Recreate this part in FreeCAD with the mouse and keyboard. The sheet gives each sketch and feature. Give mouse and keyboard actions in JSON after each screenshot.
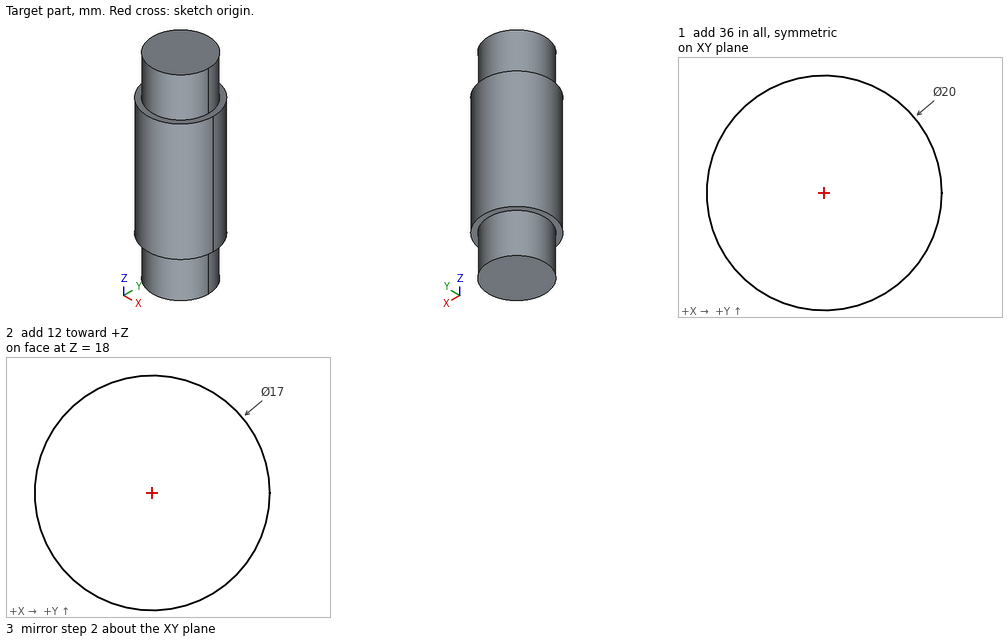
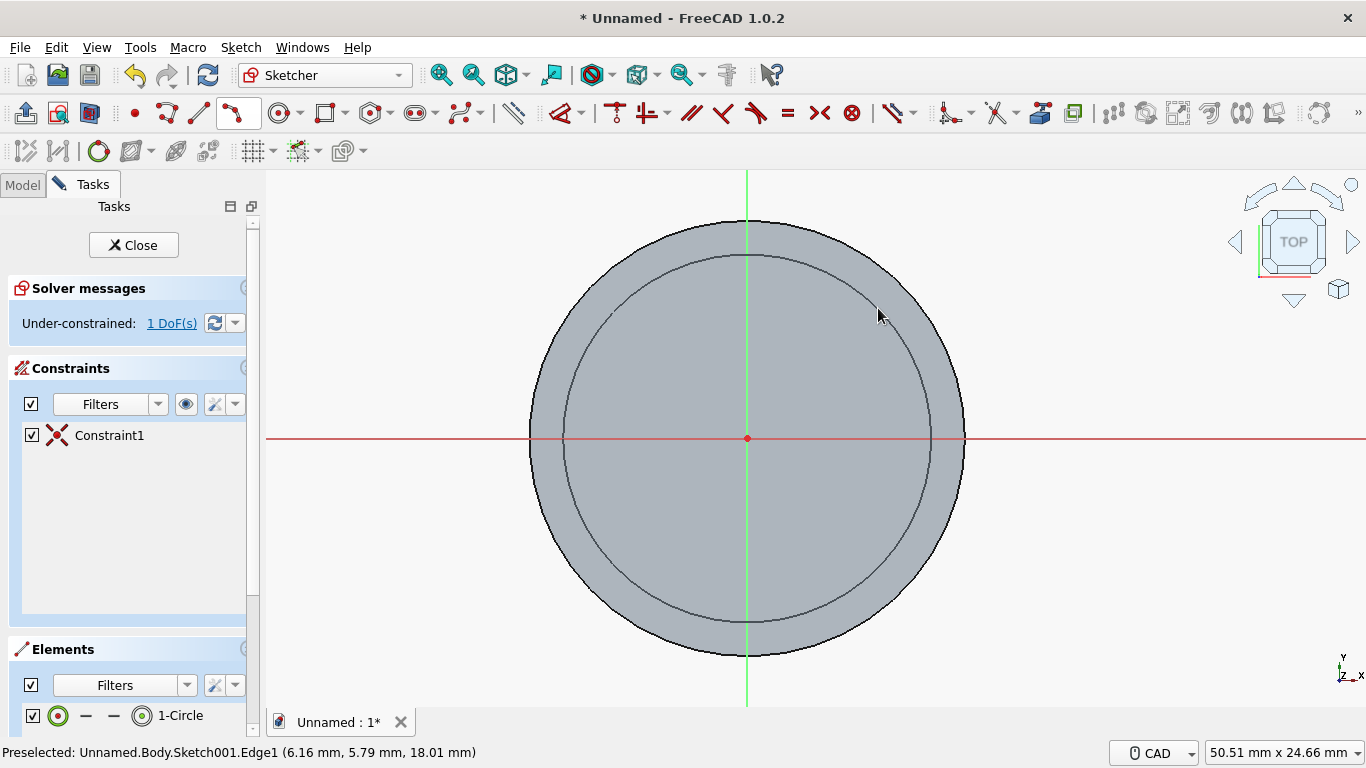
{"action": "key", "text": "d"}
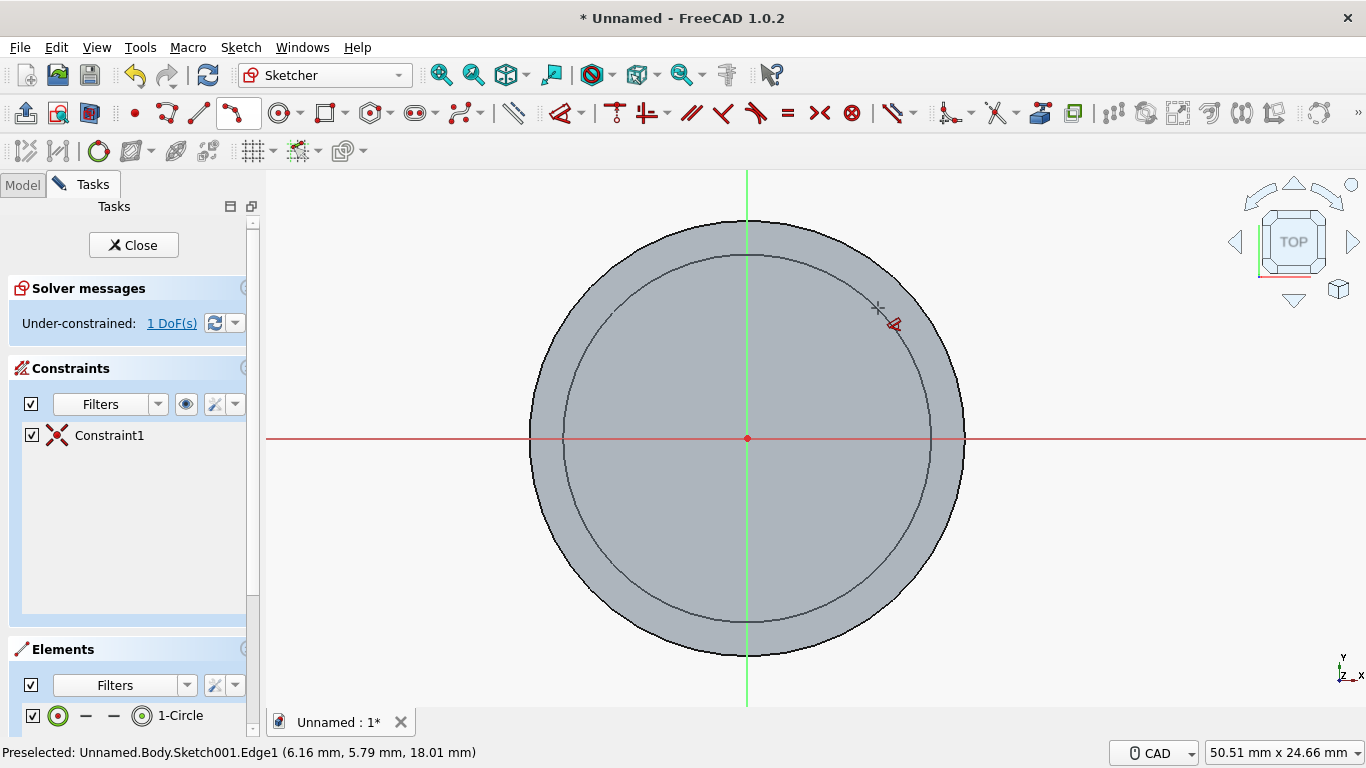
{"action": "left_click", "coordinate": [877, 308]}
{"action": "left_click", "coordinate": [900, 285]}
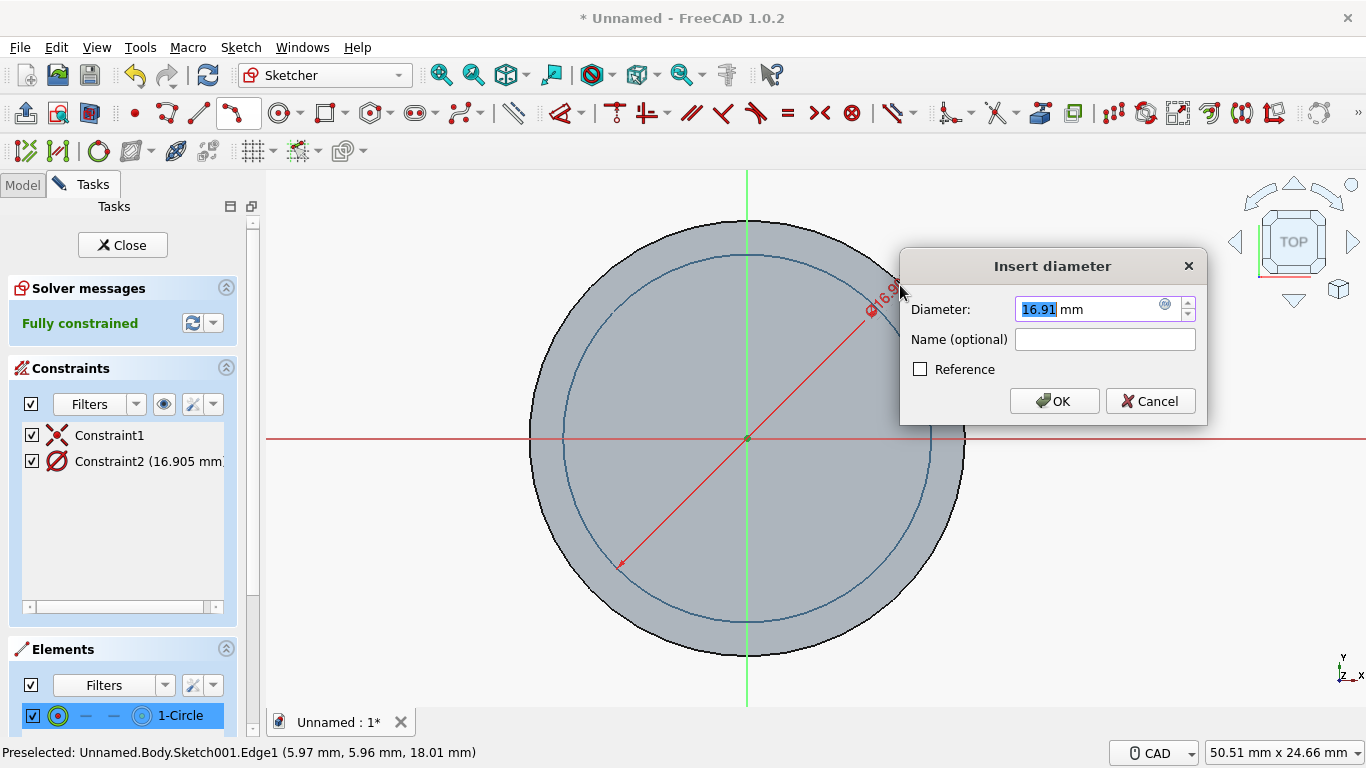
{"action": "type", "text": "17"}
{"action": "key", "text": "Return"}
{"action": "key", "text": "Escape"}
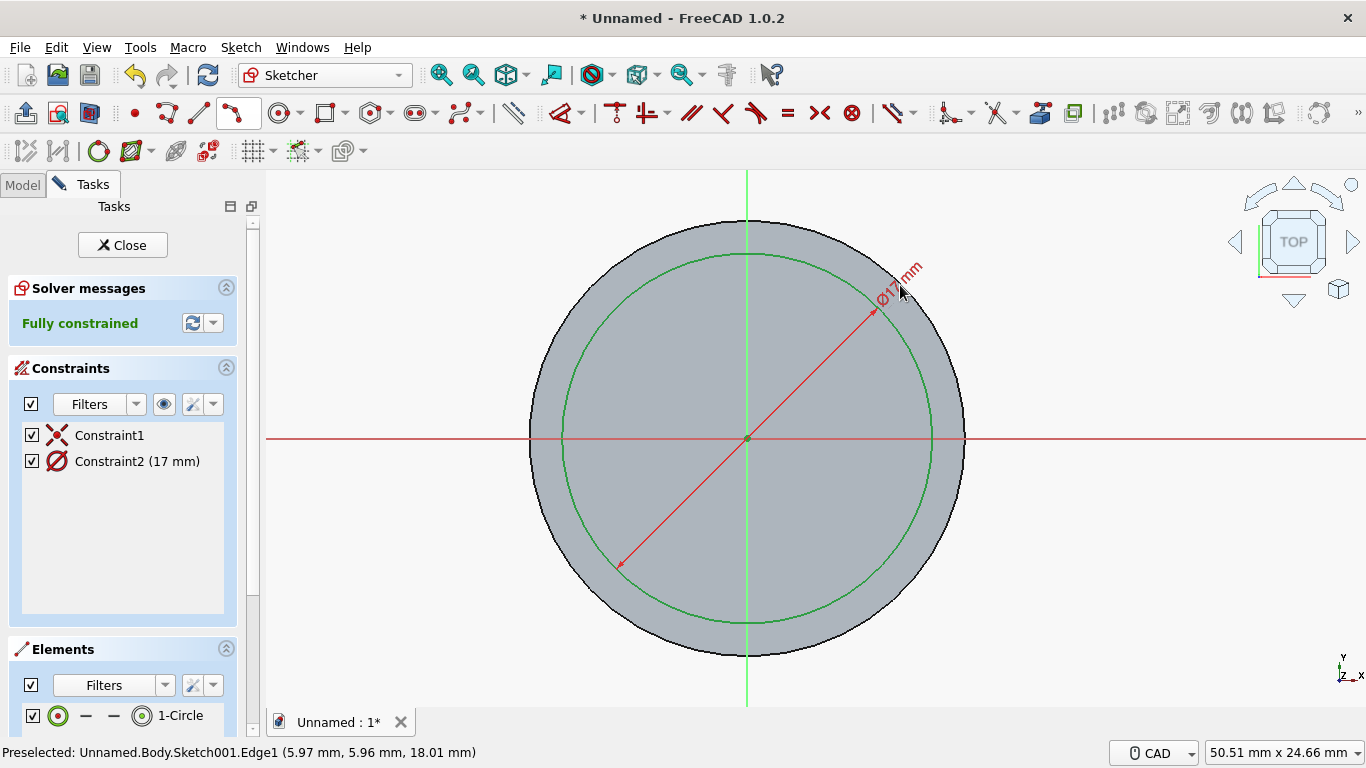
{"action": "left_click", "coordinate": [123, 245]}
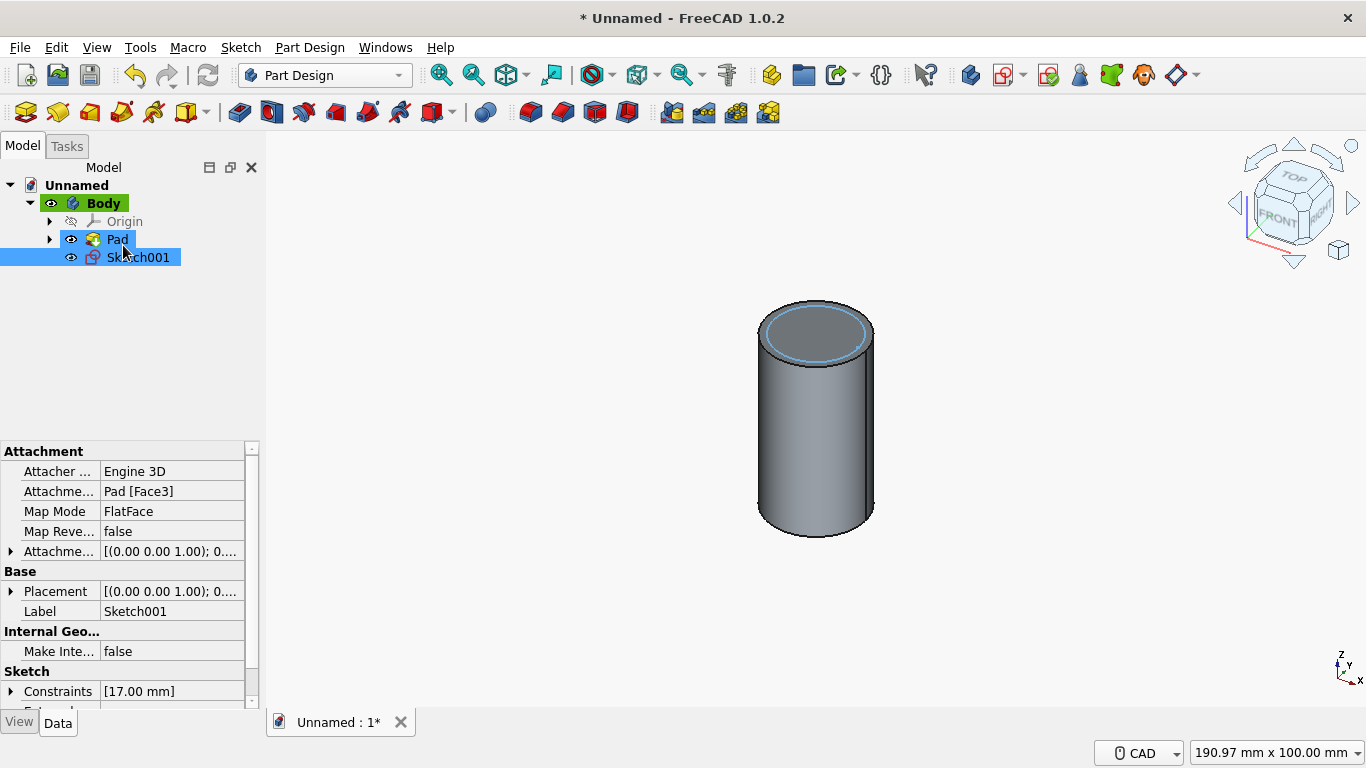
{"action": "left_click", "coordinate": [26, 112]}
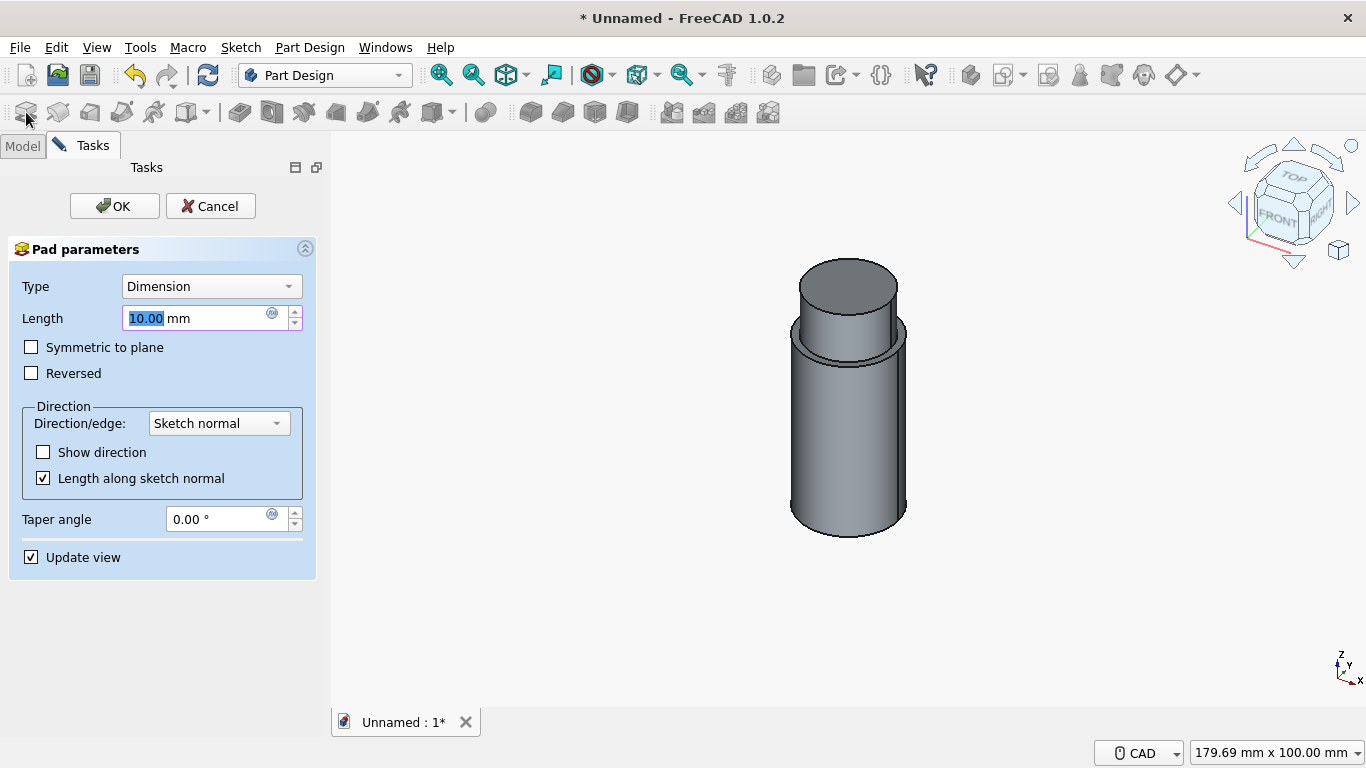
{"action": "type", "text": "12"}
{"action": "key", "text": "Tab"}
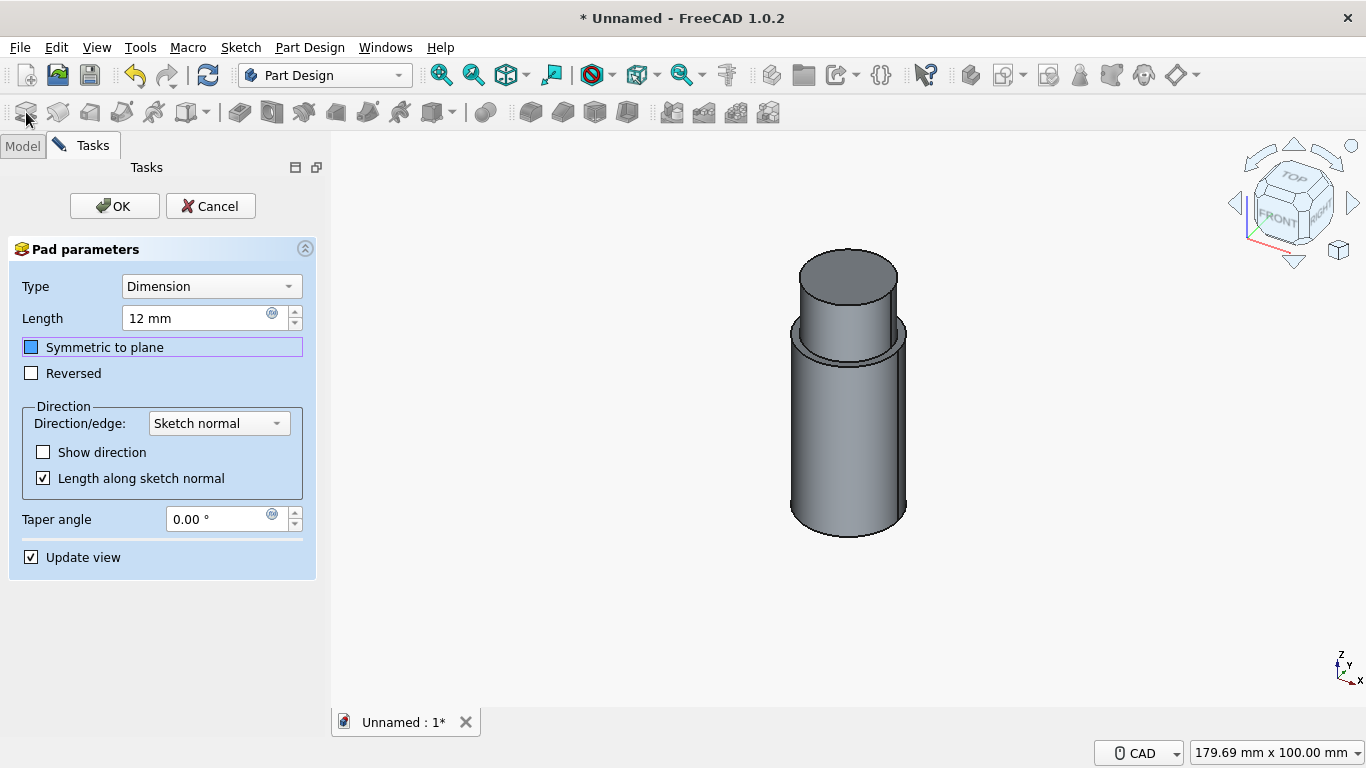
{"action": "left_click", "coordinate": [115, 206]}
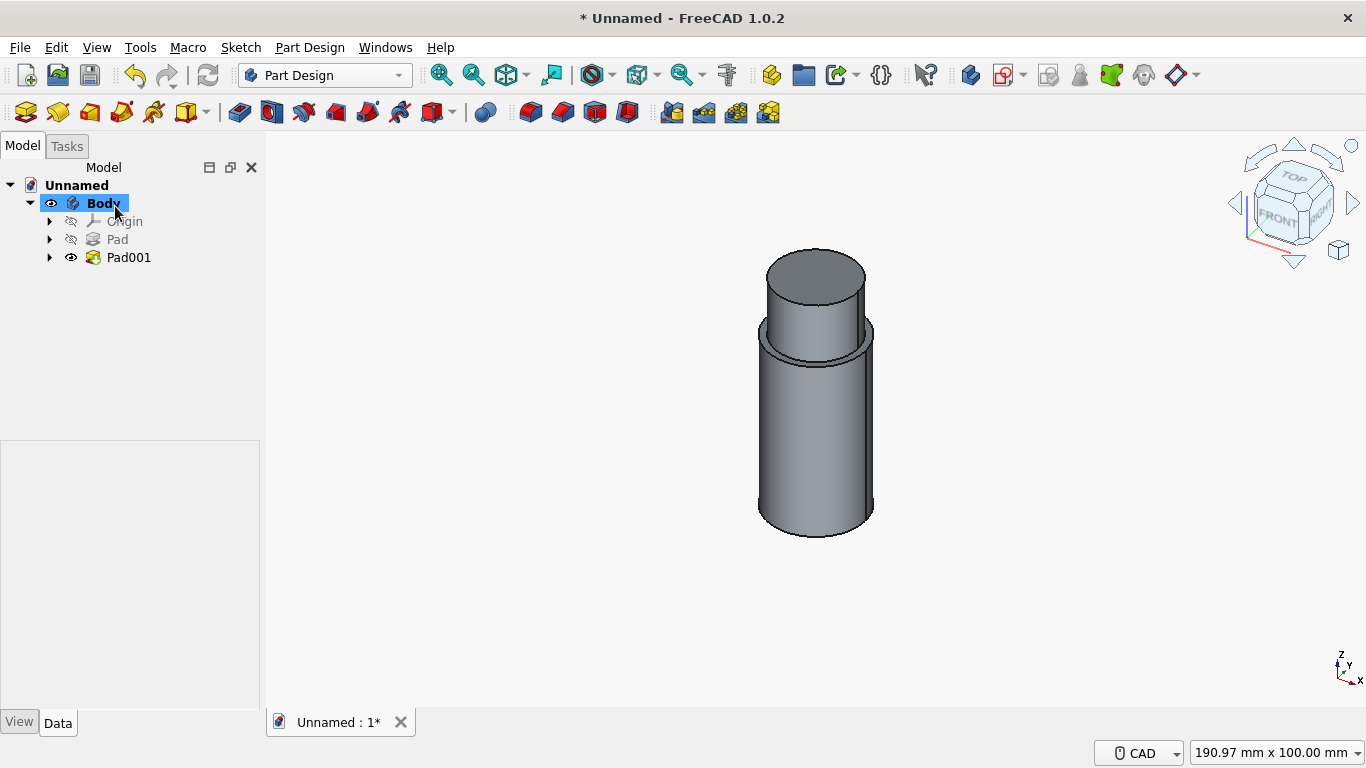
{"action": "left_click", "coordinate": [116, 257]}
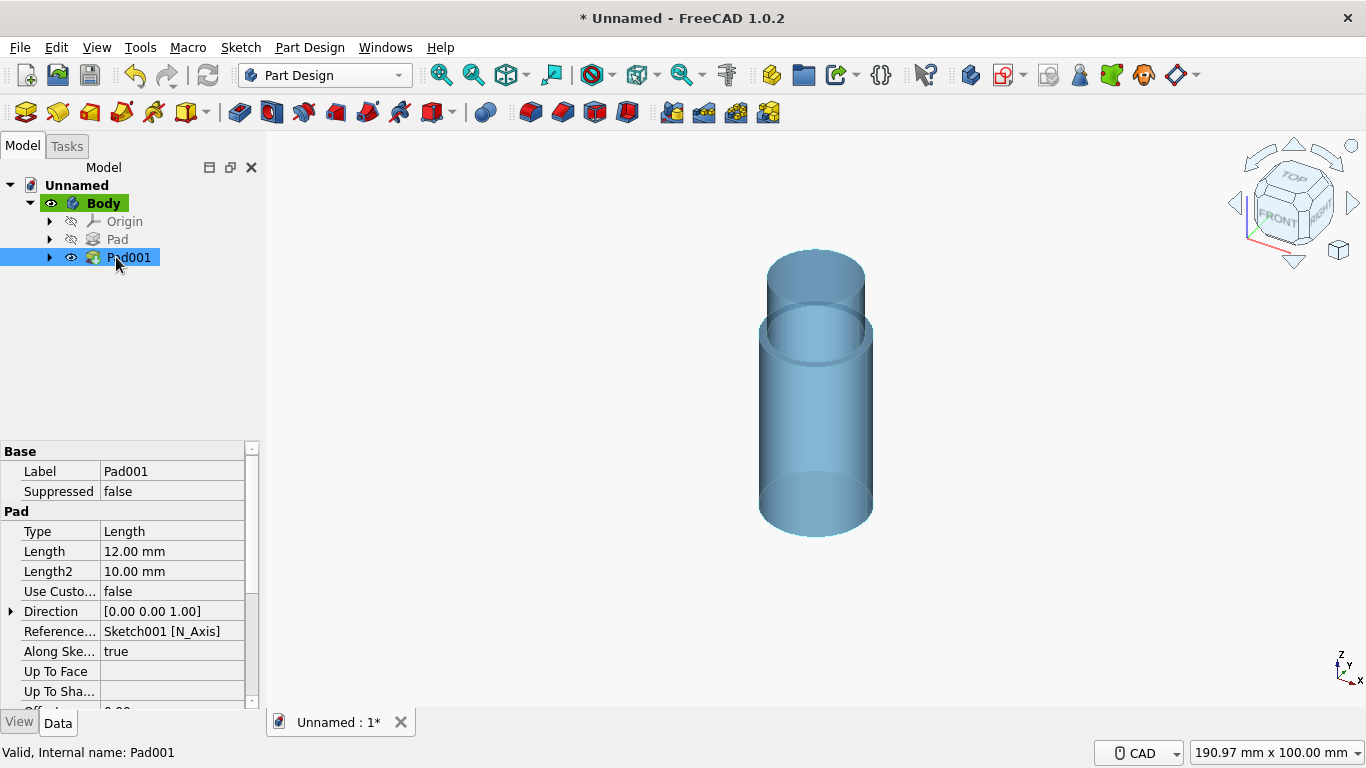
{"action": "left_click", "coordinate": [672, 112]}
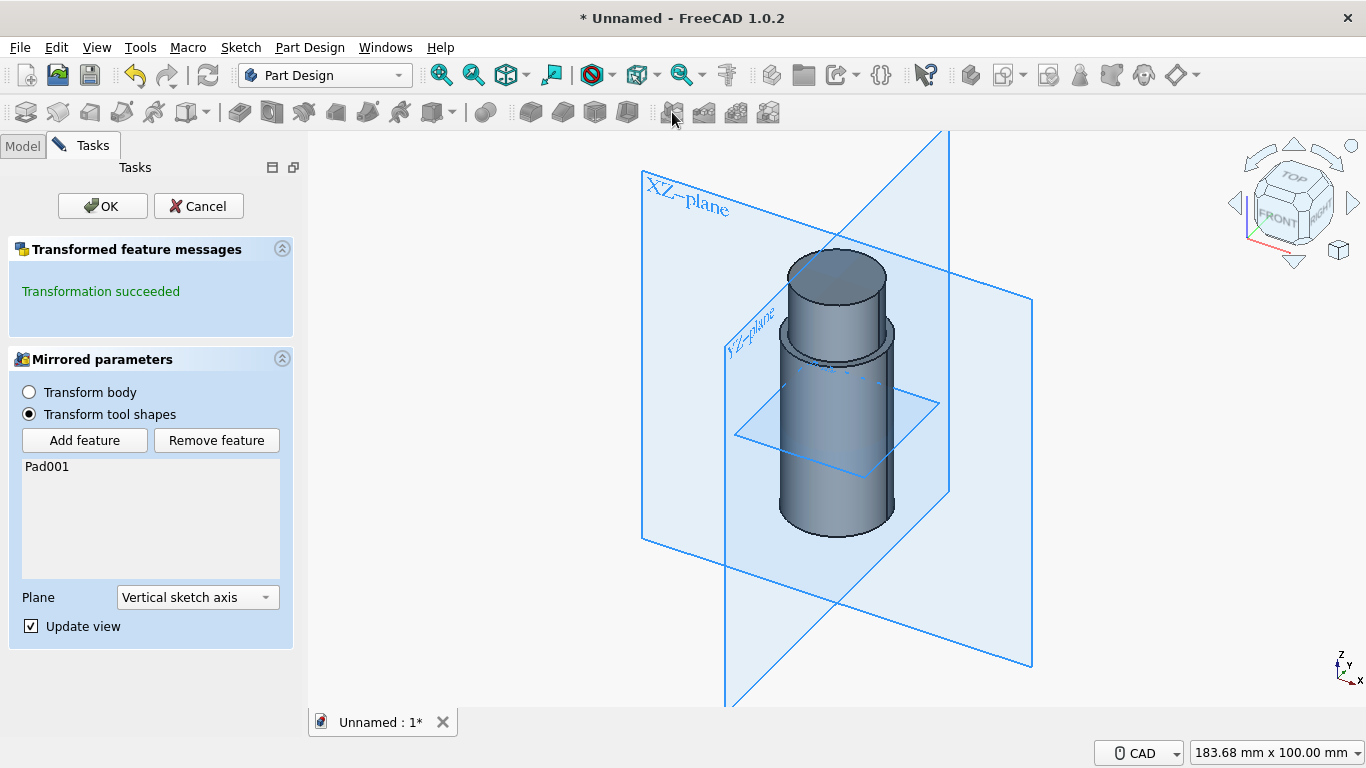
{"action": "left_click", "coordinate": [198, 598]}